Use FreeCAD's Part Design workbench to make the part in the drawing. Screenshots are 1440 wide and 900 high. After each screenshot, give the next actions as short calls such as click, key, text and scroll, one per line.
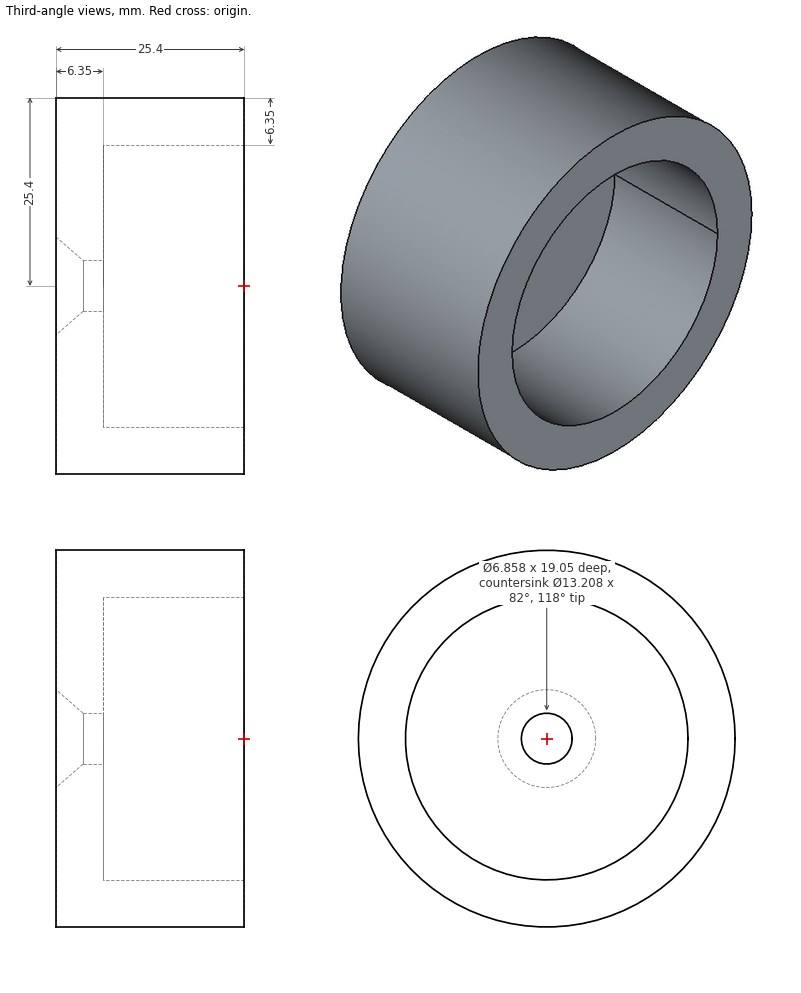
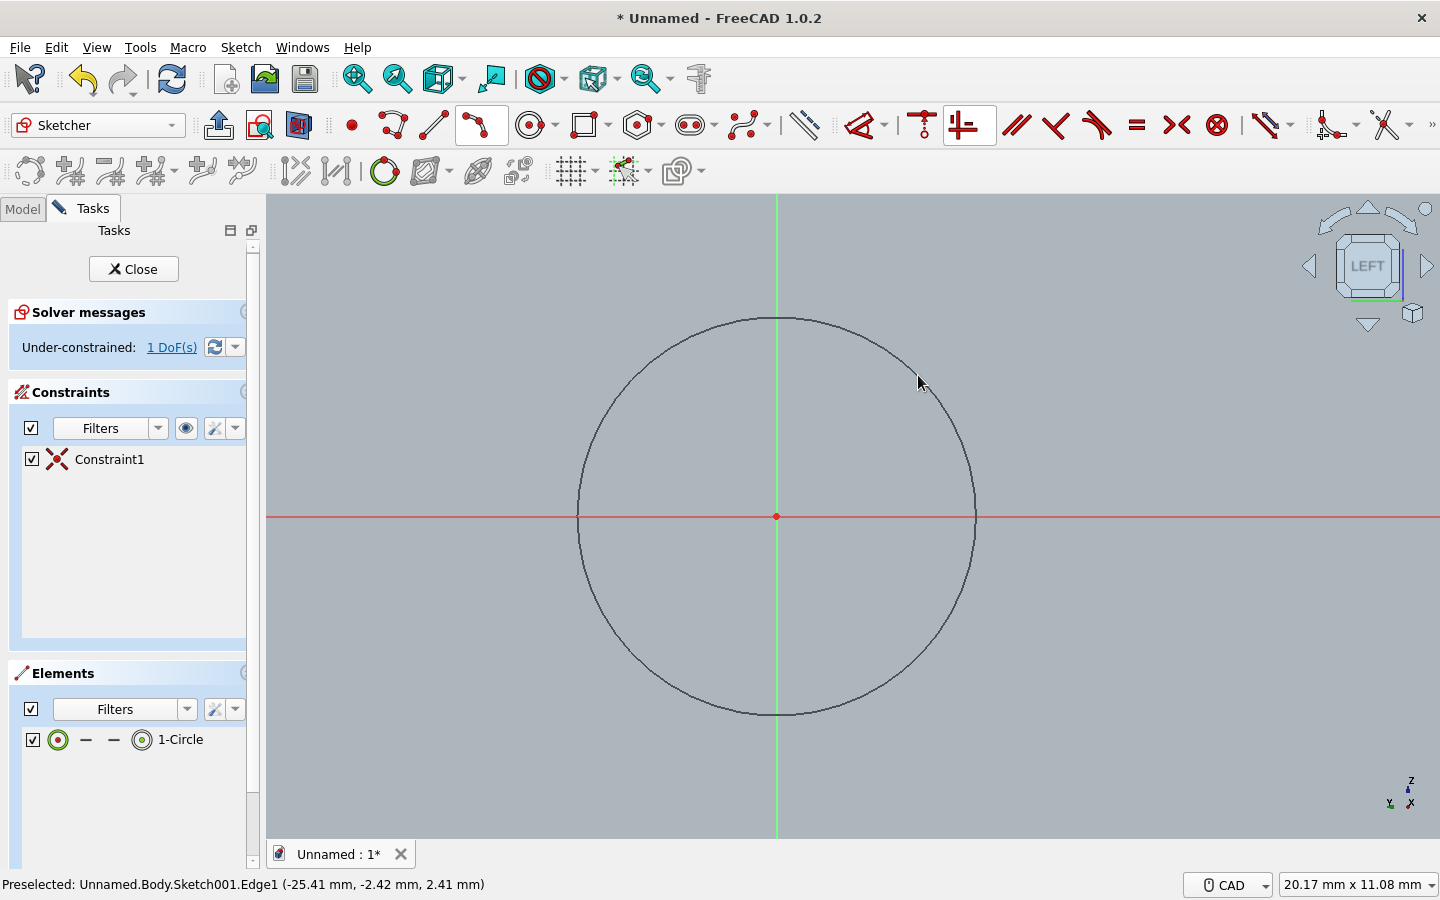
click(860, 126)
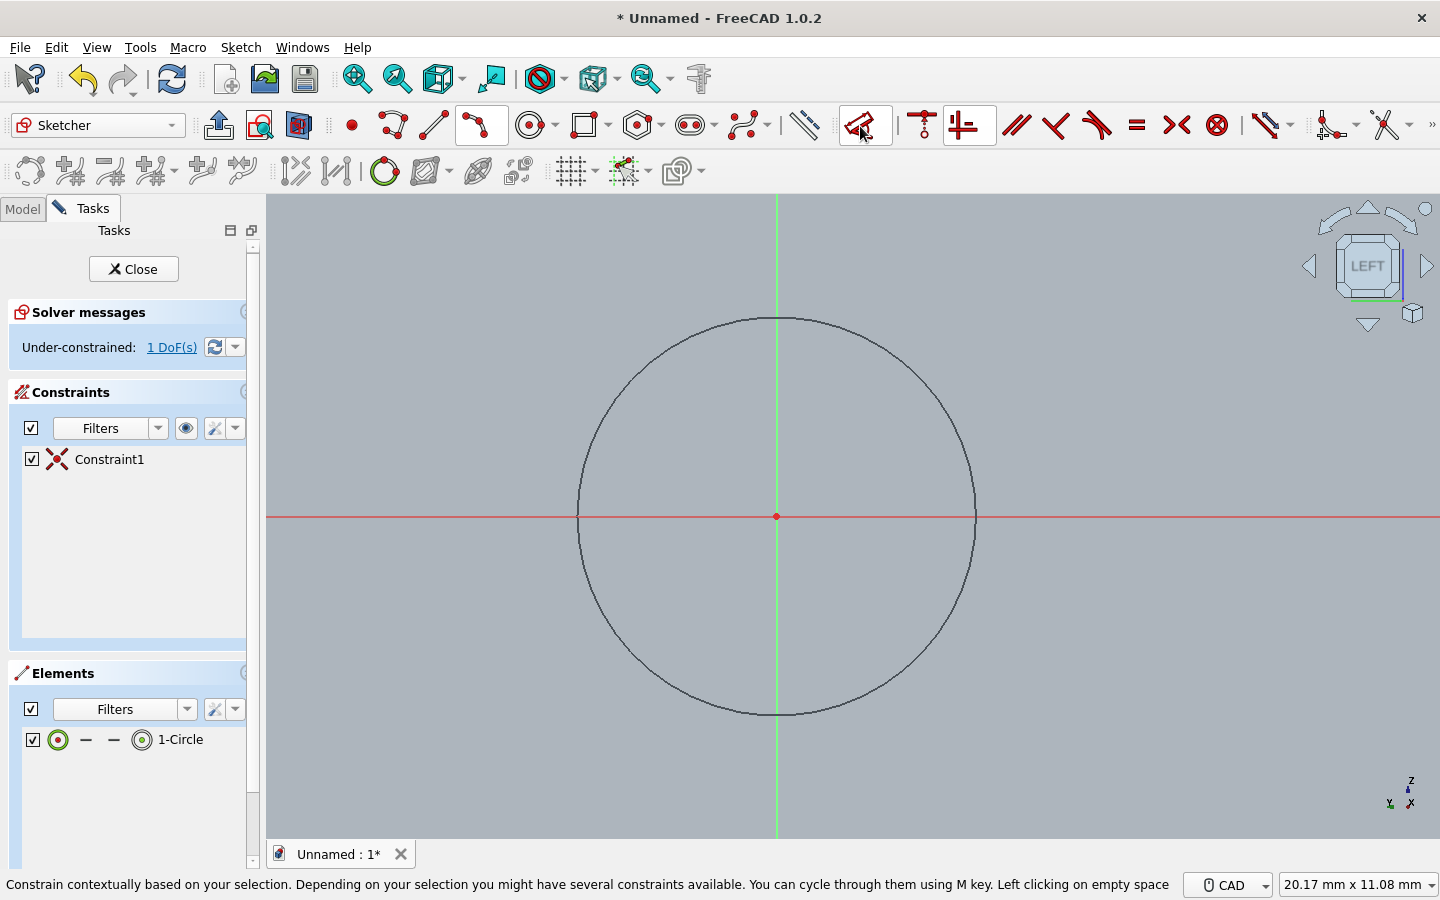
click(917, 375)
click(940, 352)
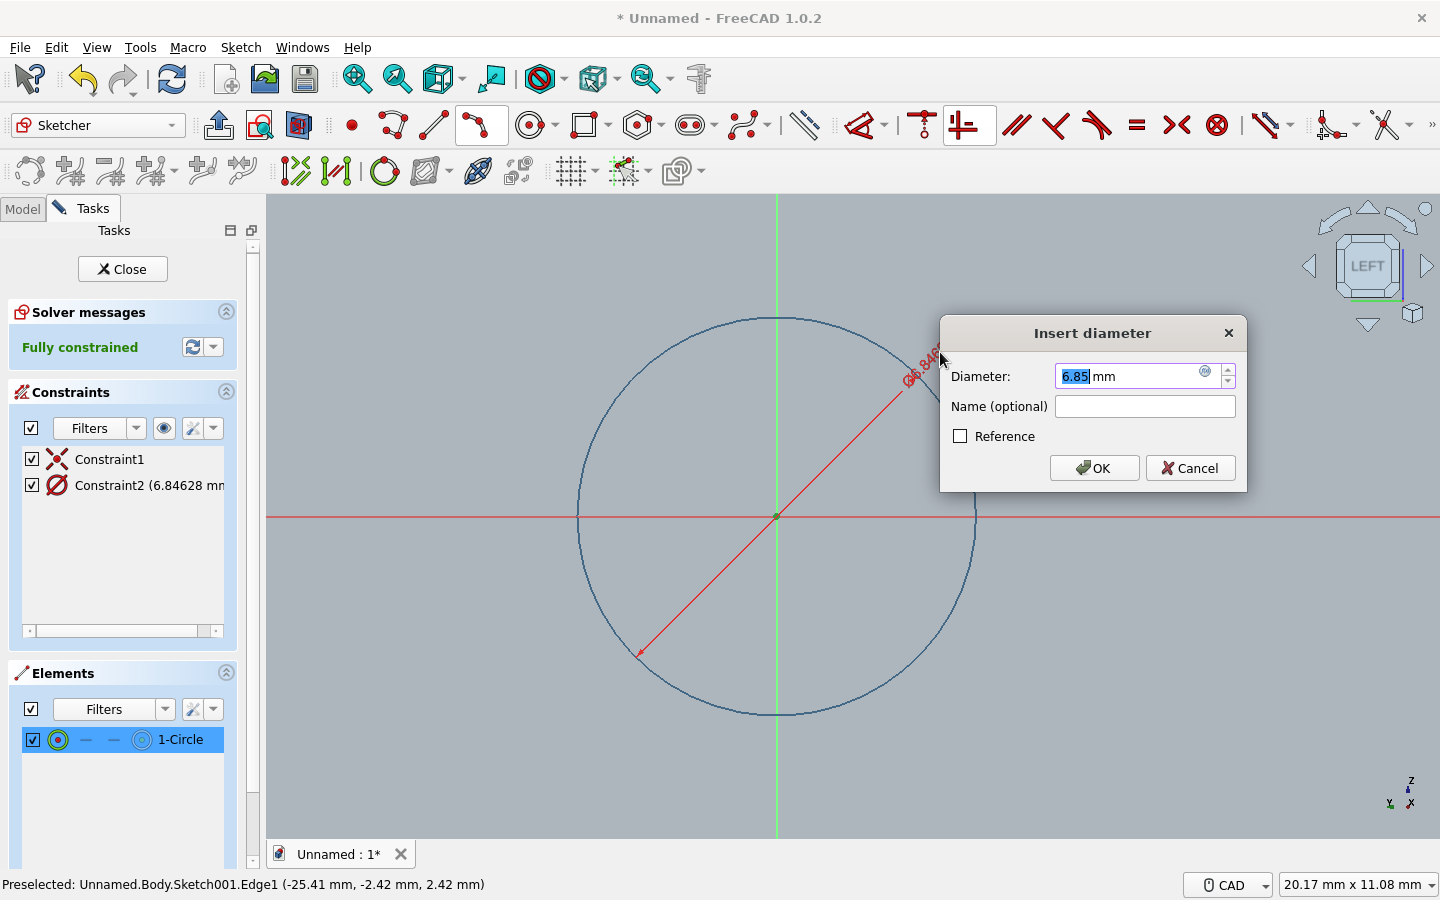
text(6.858)
key(Return)
key(Escape)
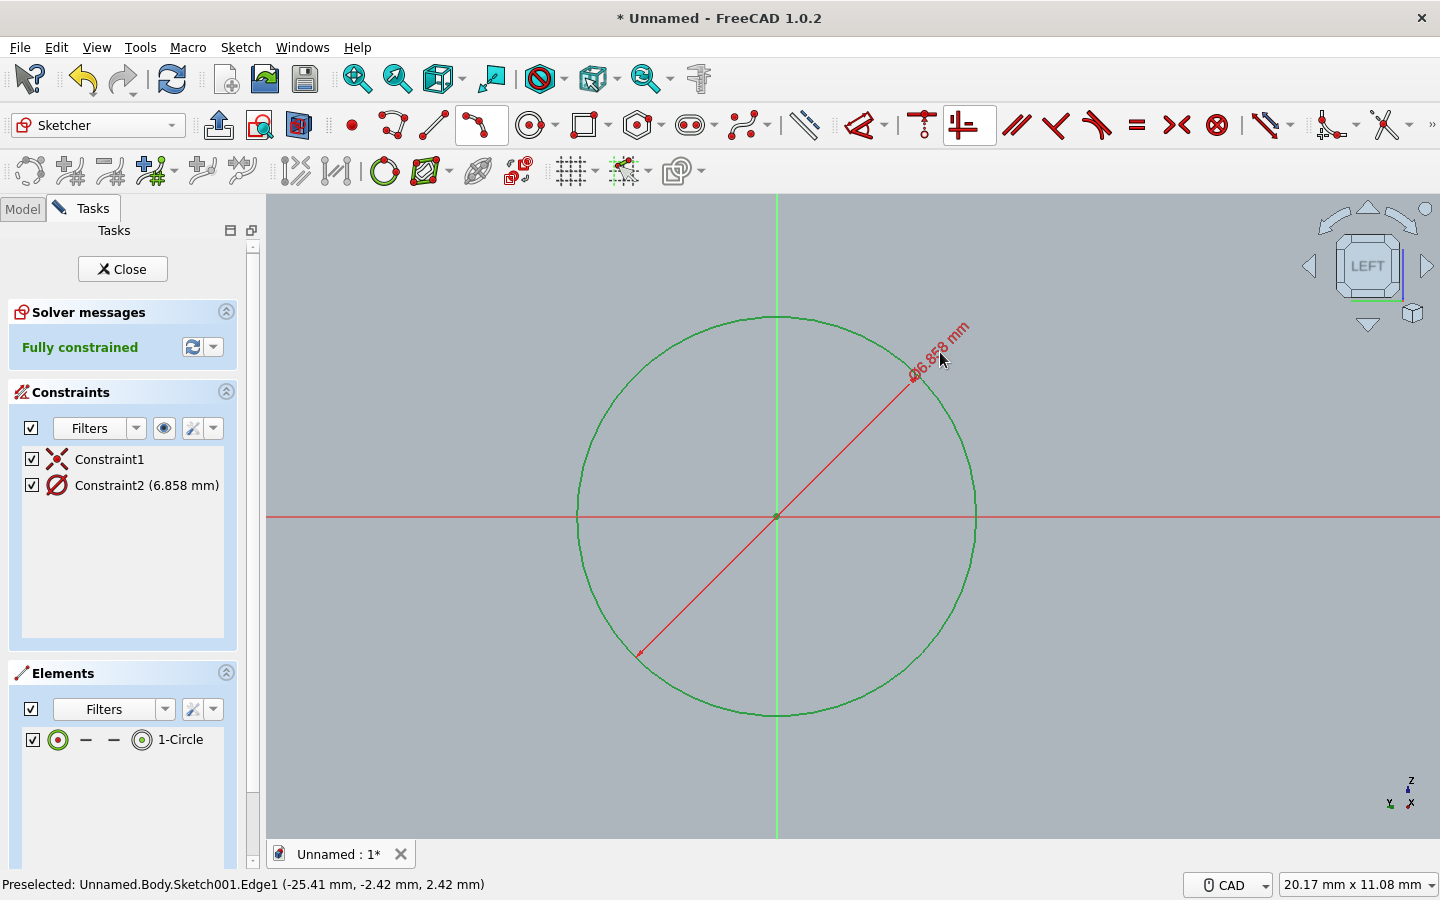
click(123, 269)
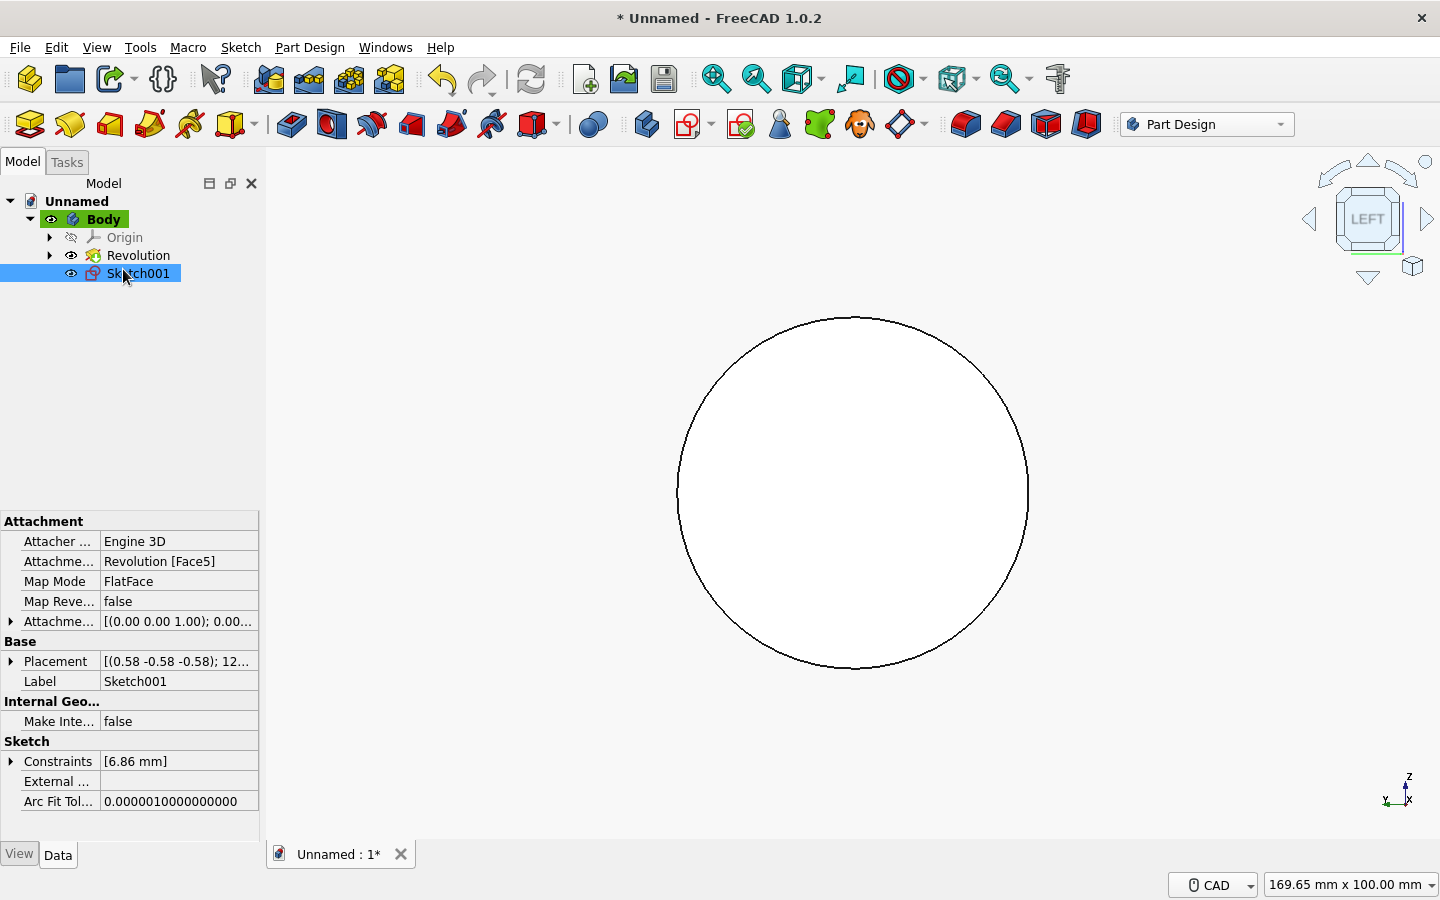
click(332, 124)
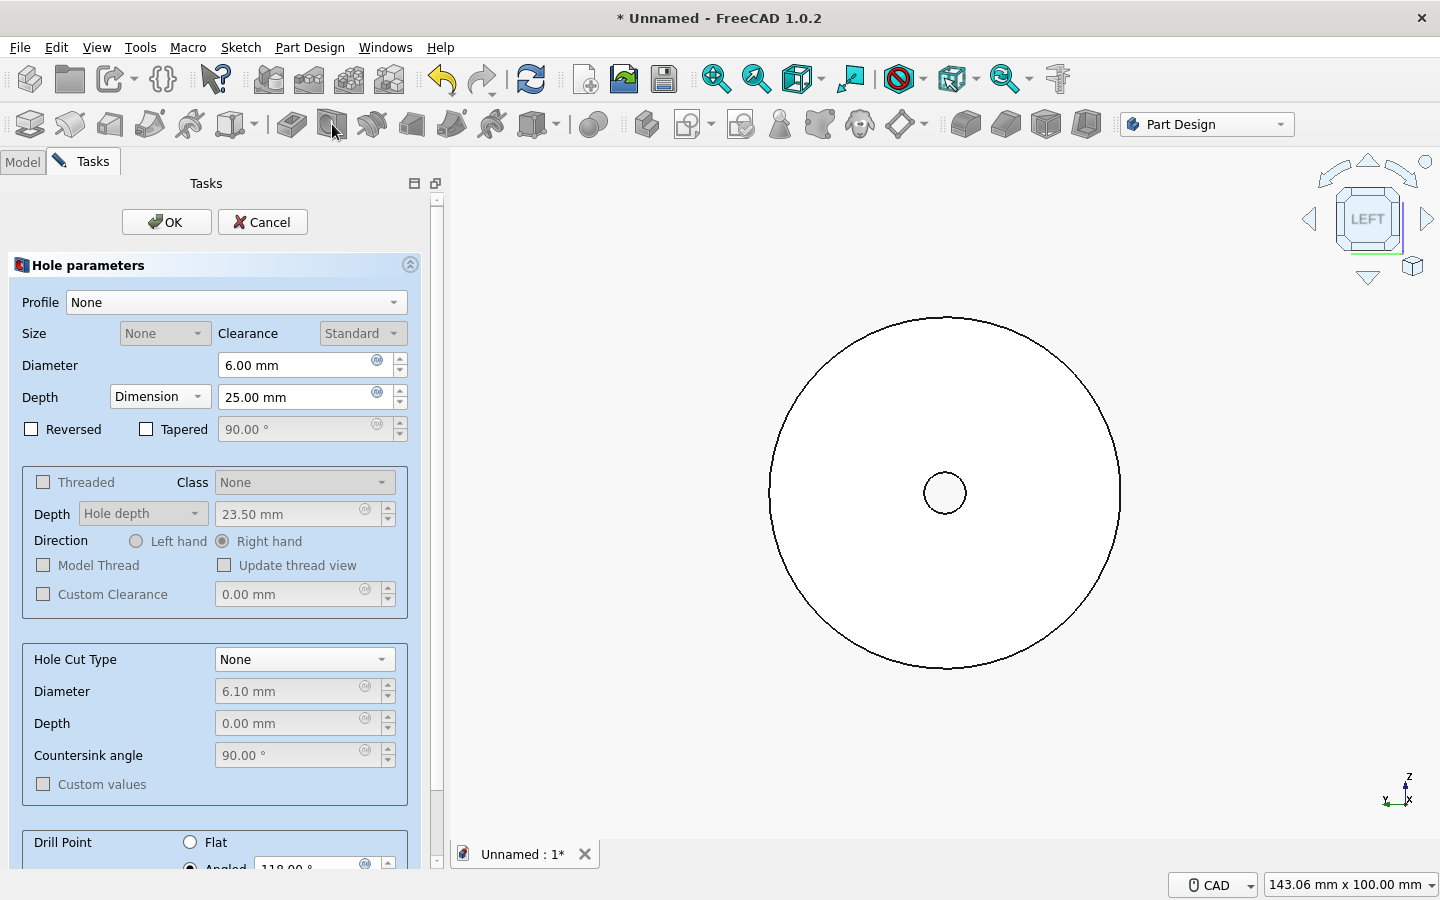
triple_click(305, 365)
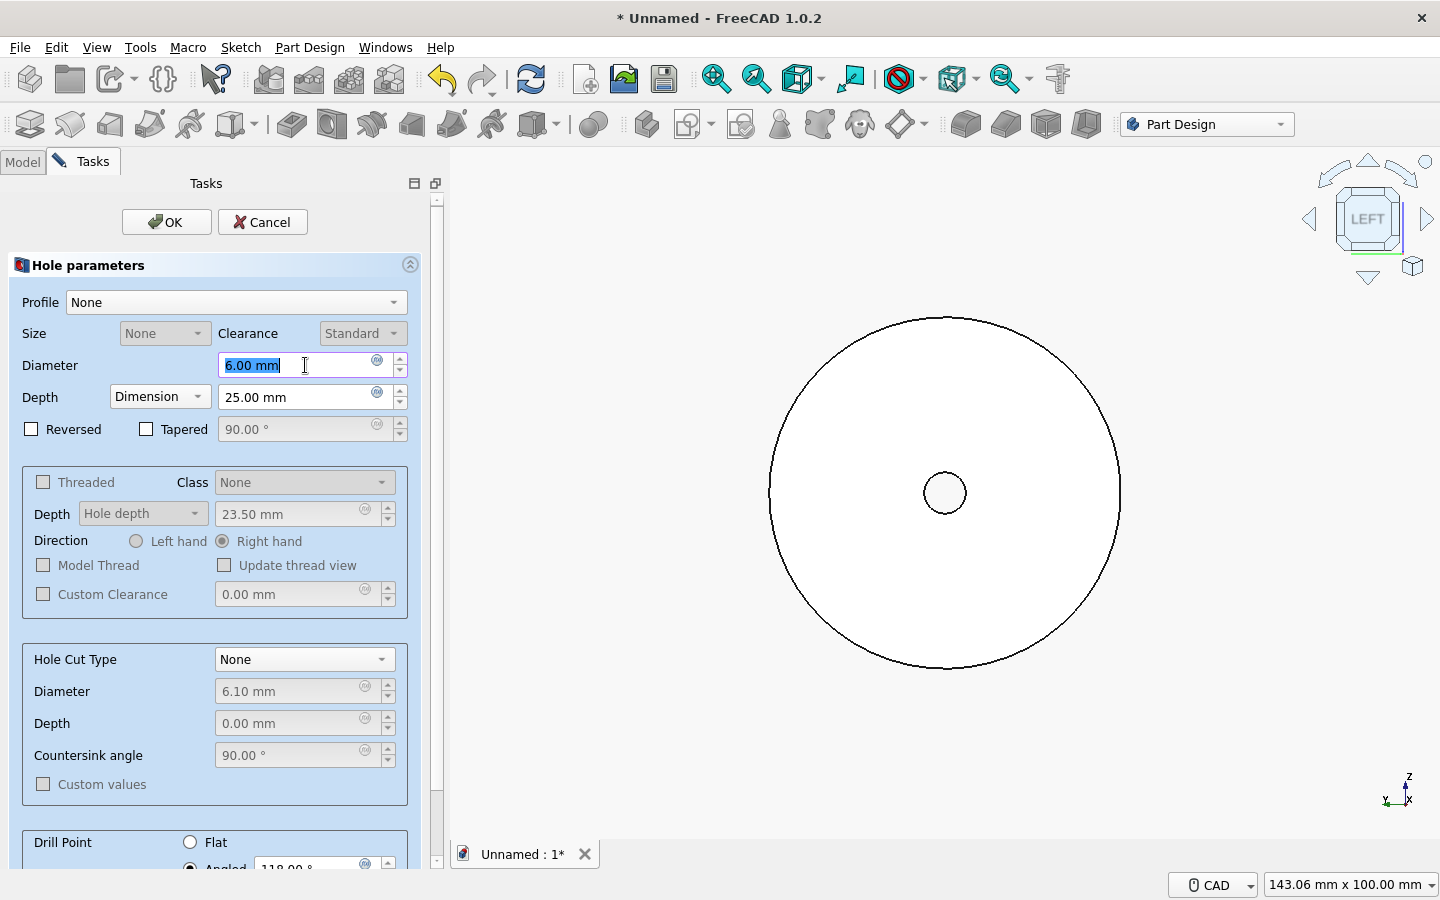
text(6.858)
key(Tab)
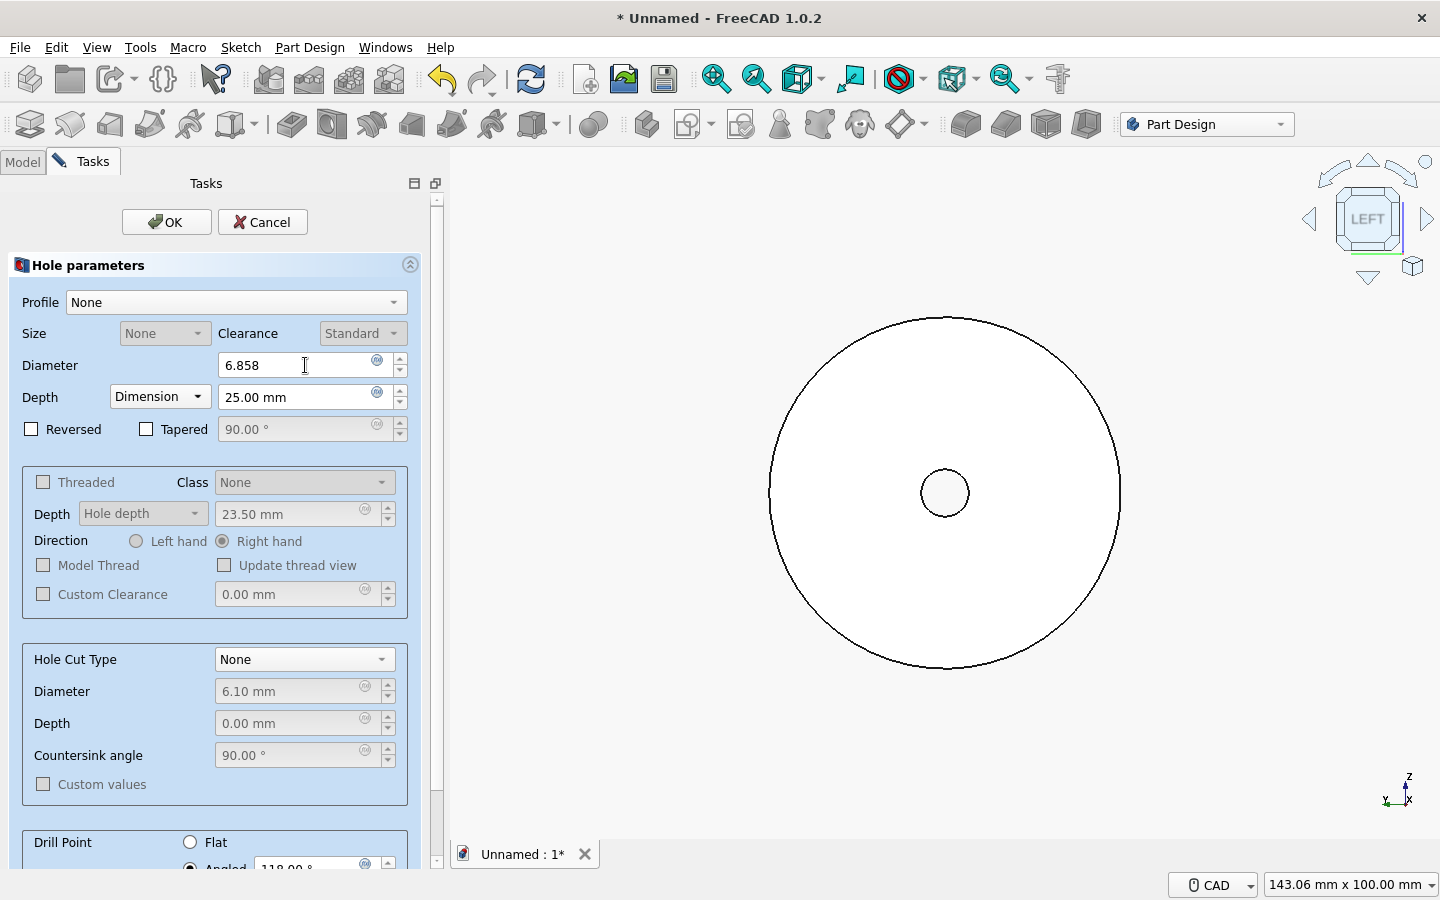
triple_click(305, 397)